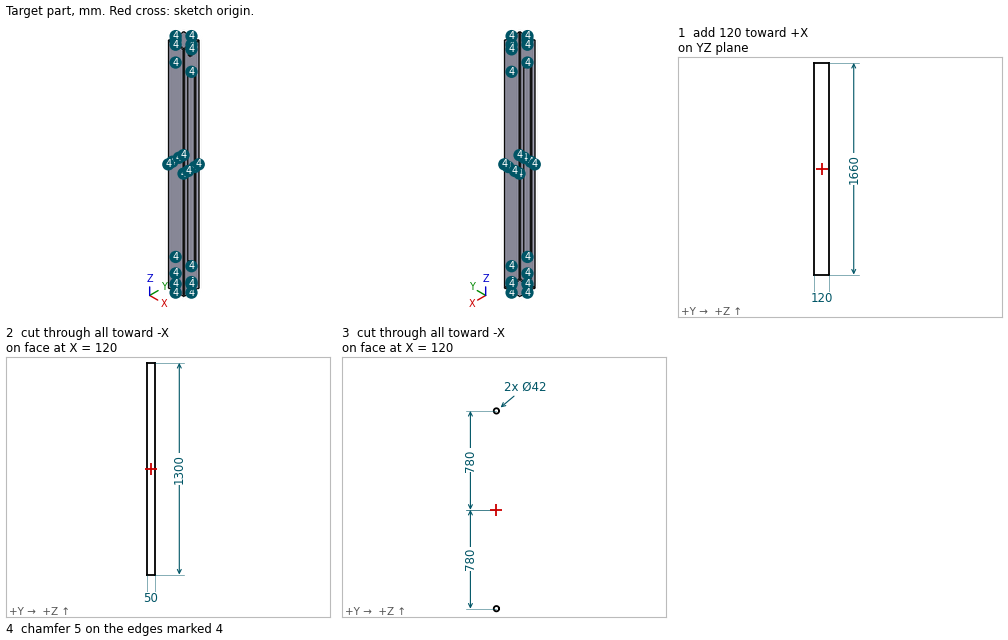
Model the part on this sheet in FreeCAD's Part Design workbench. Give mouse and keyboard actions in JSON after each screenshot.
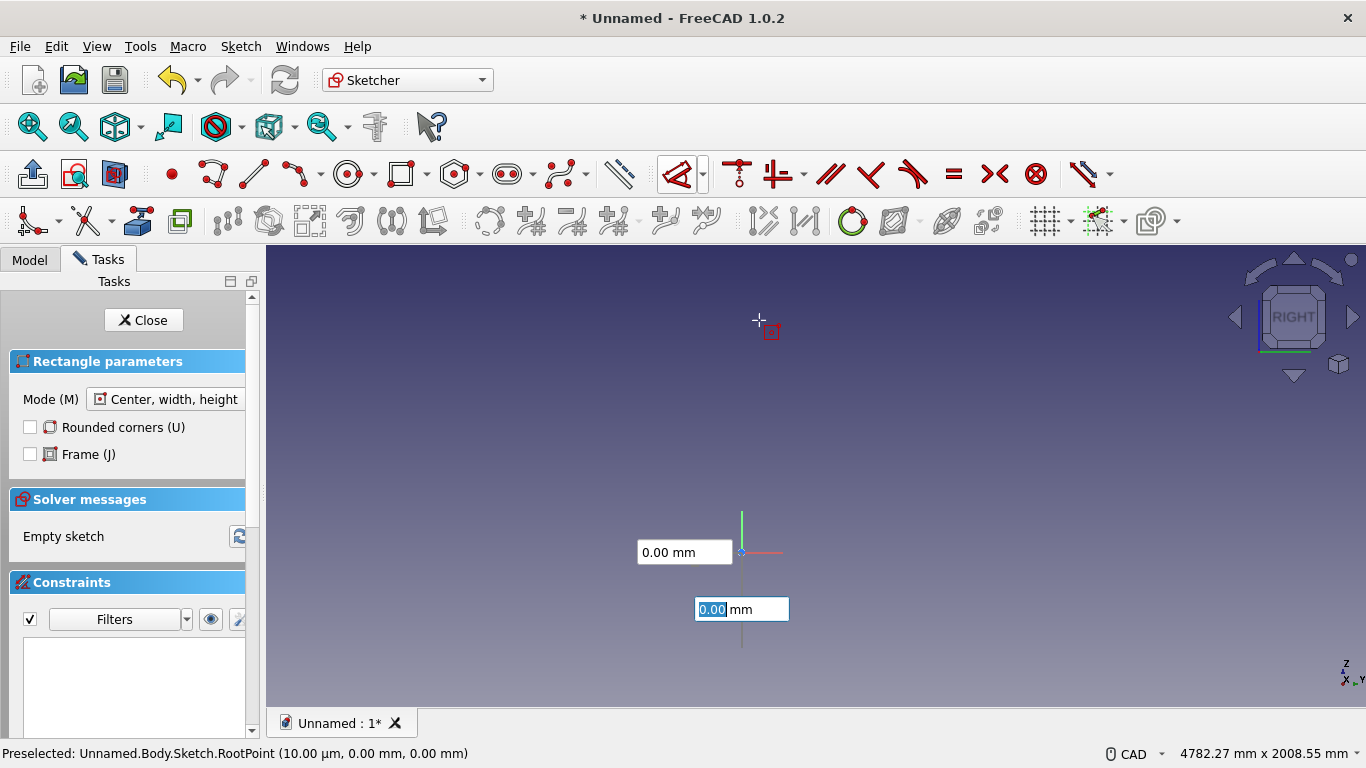
{"action": "left_click", "coordinate": [759, 320]}
{"action": "key", "text": "Escape"}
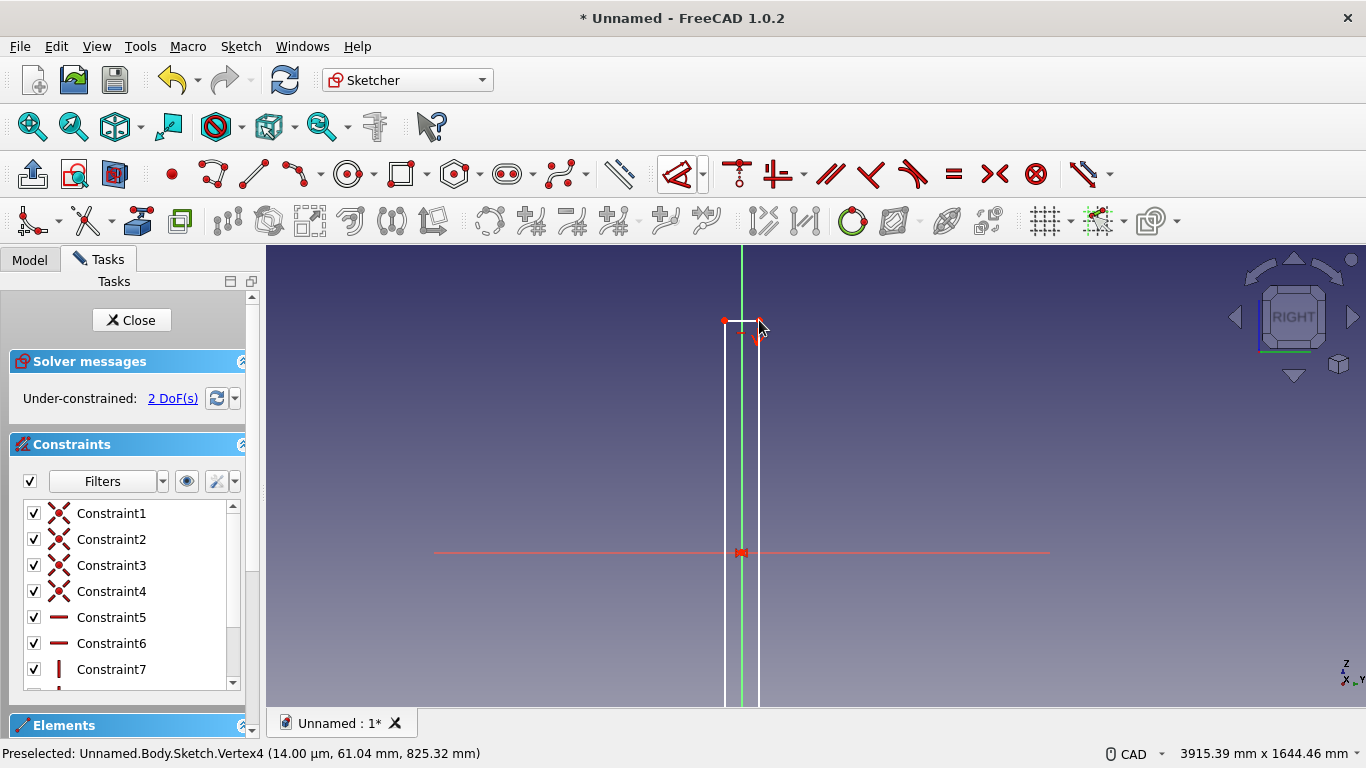
{"action": "key", "text": "d"}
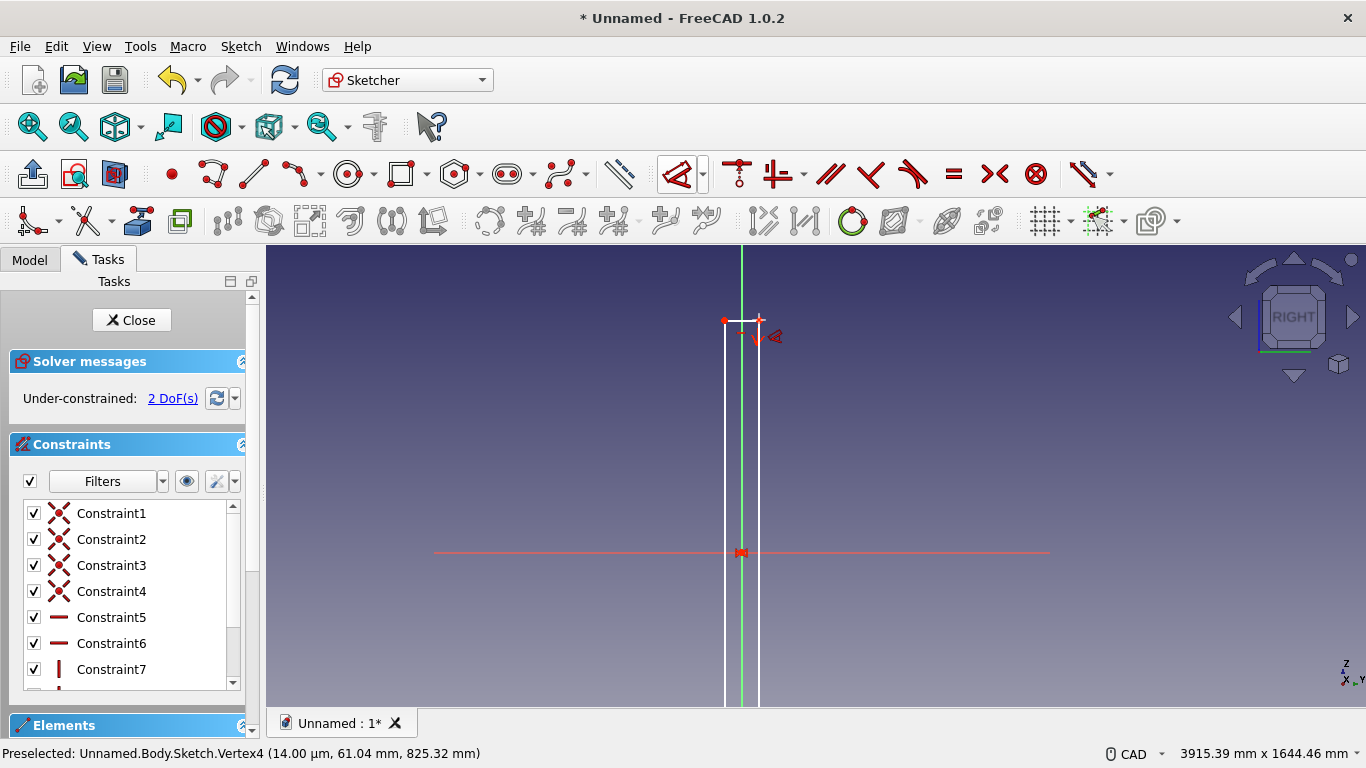
{"action": "scroll", "coordinate": [759, 320], "scroll_direction": "down", "scroll_amount": 2}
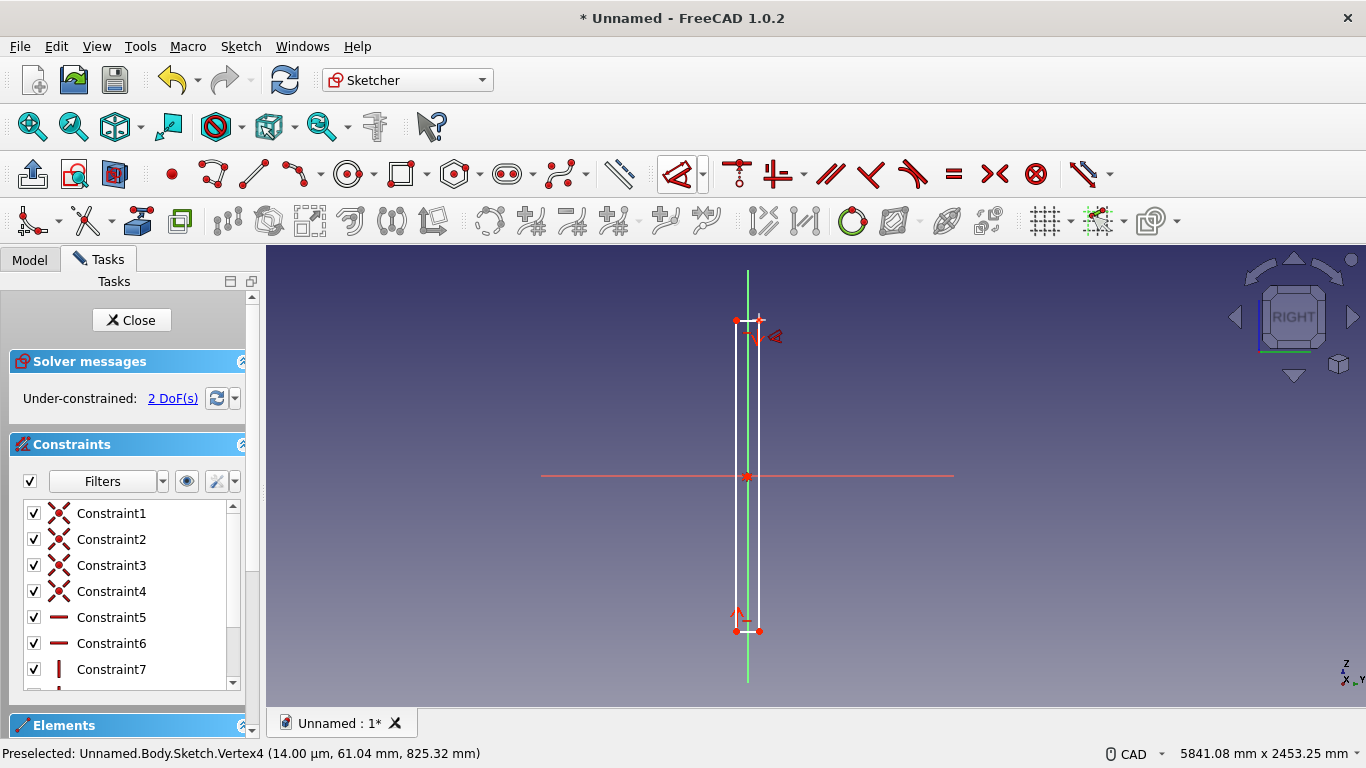
{"action": "scroll", "coordinate": [745, 632], "scroll_direction": "up", "scroll_amount": 3}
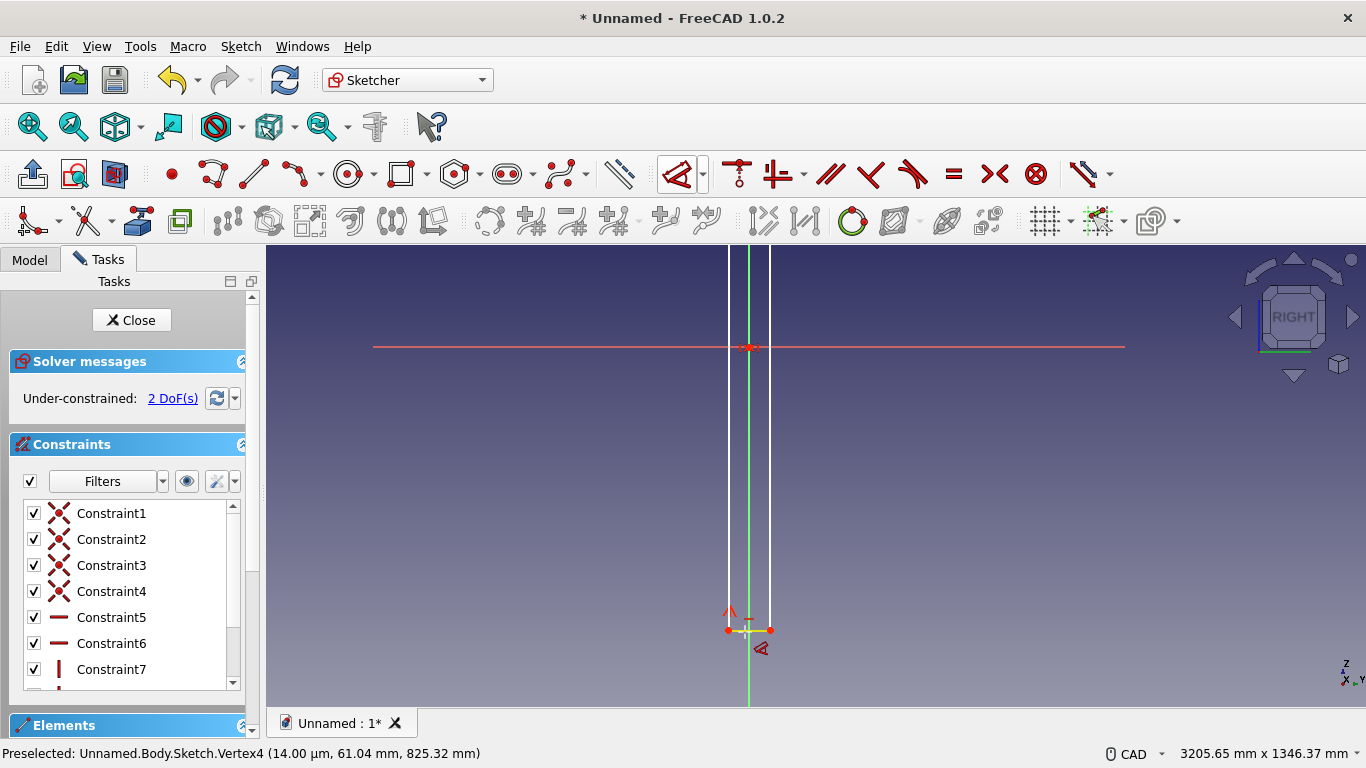
{"action": "left_click", "coordinate": [745, 631]}
{"action": "left_click", "coordinate": [735, 665]}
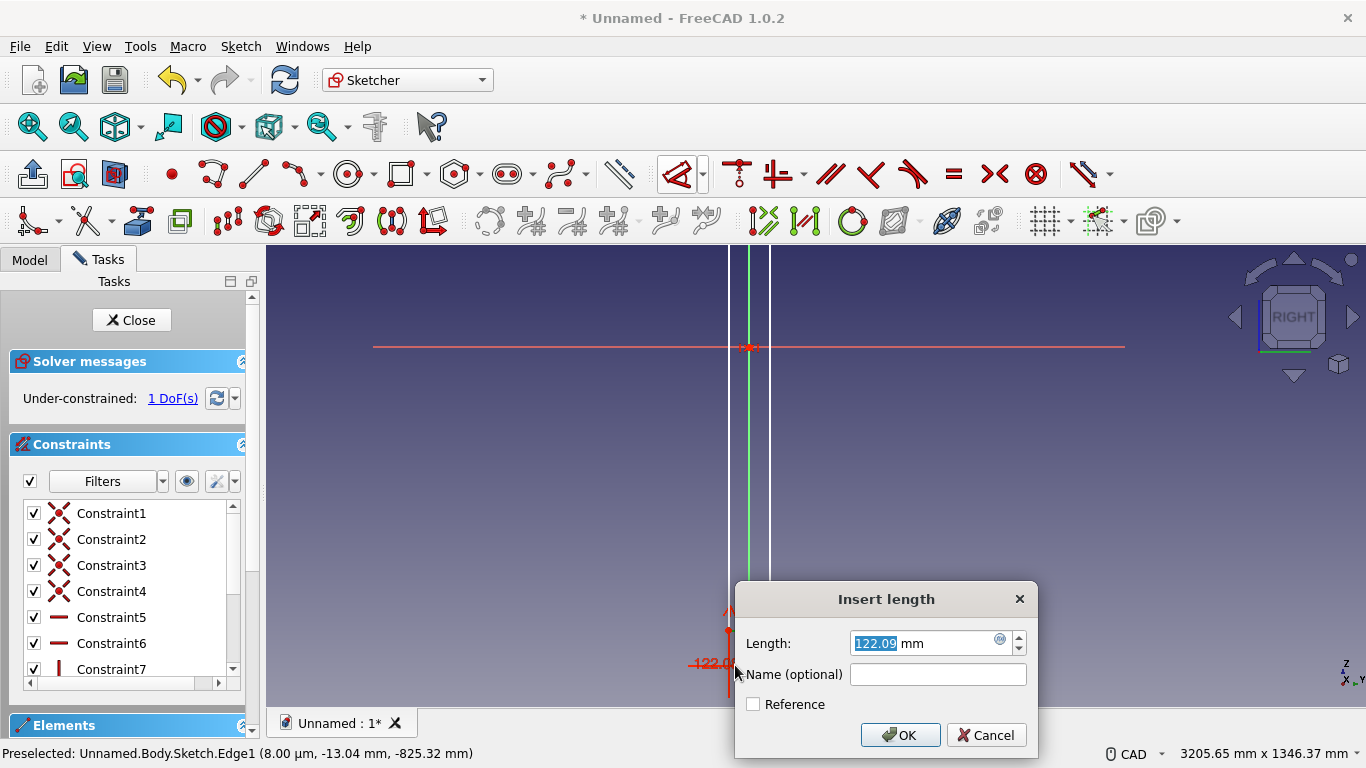
{"action": "type", "text": "120"}
{"action": "key", "text": "Return"}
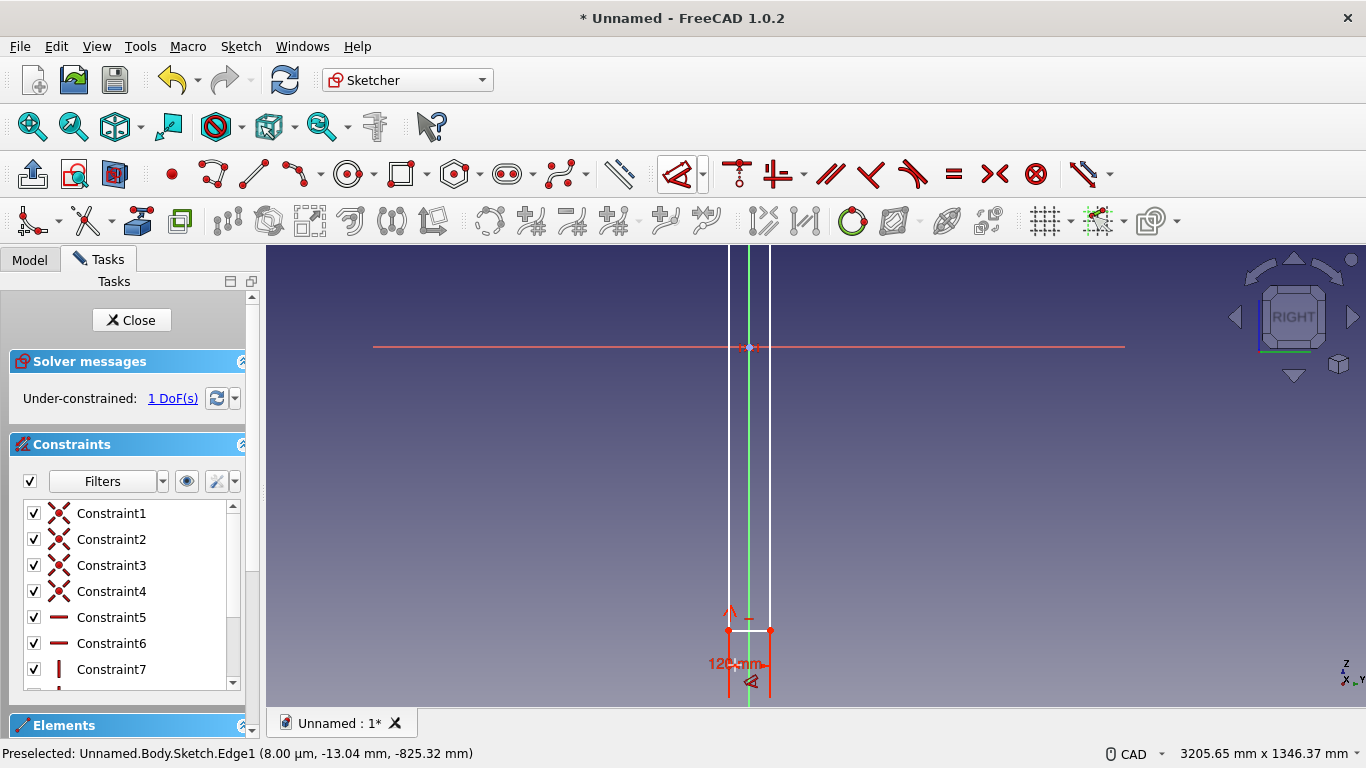
{"action": "left_click", "coordinate": [770, 461]}
{"action": "left_click", "coordinate": [804, 452]}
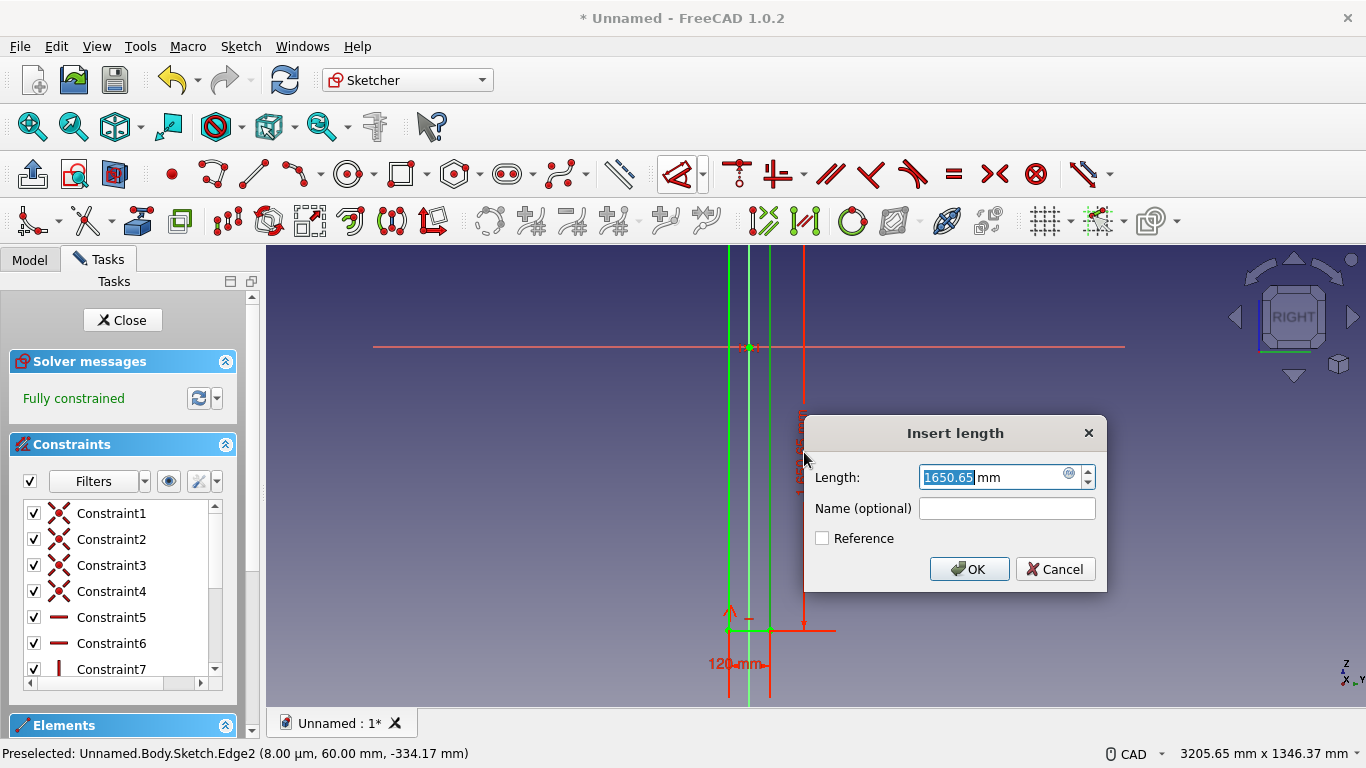
{"action": "type", "text": "1660"}
{"action": "key", "text": "Return"}
{"action": "key", "text": "Escape"}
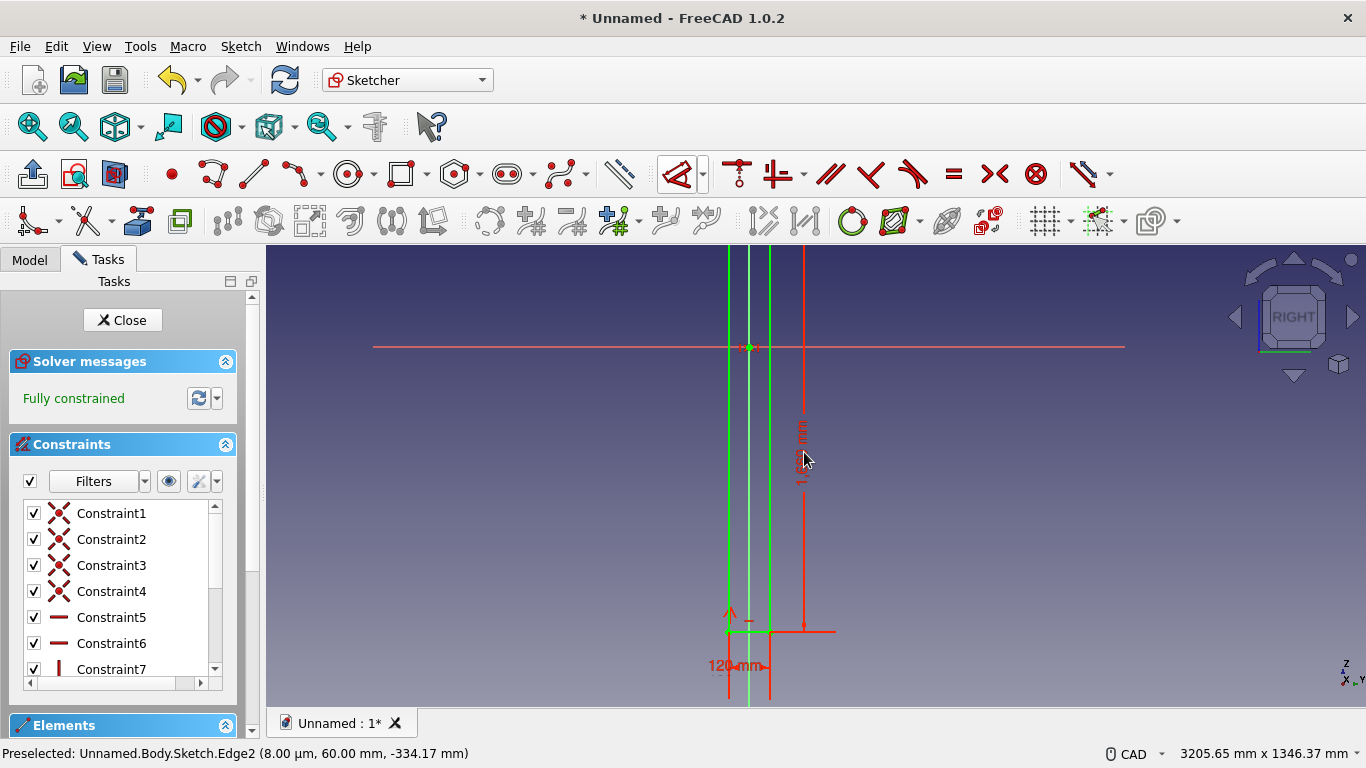
{"action": "left_click", "coordinate": [123, 320]}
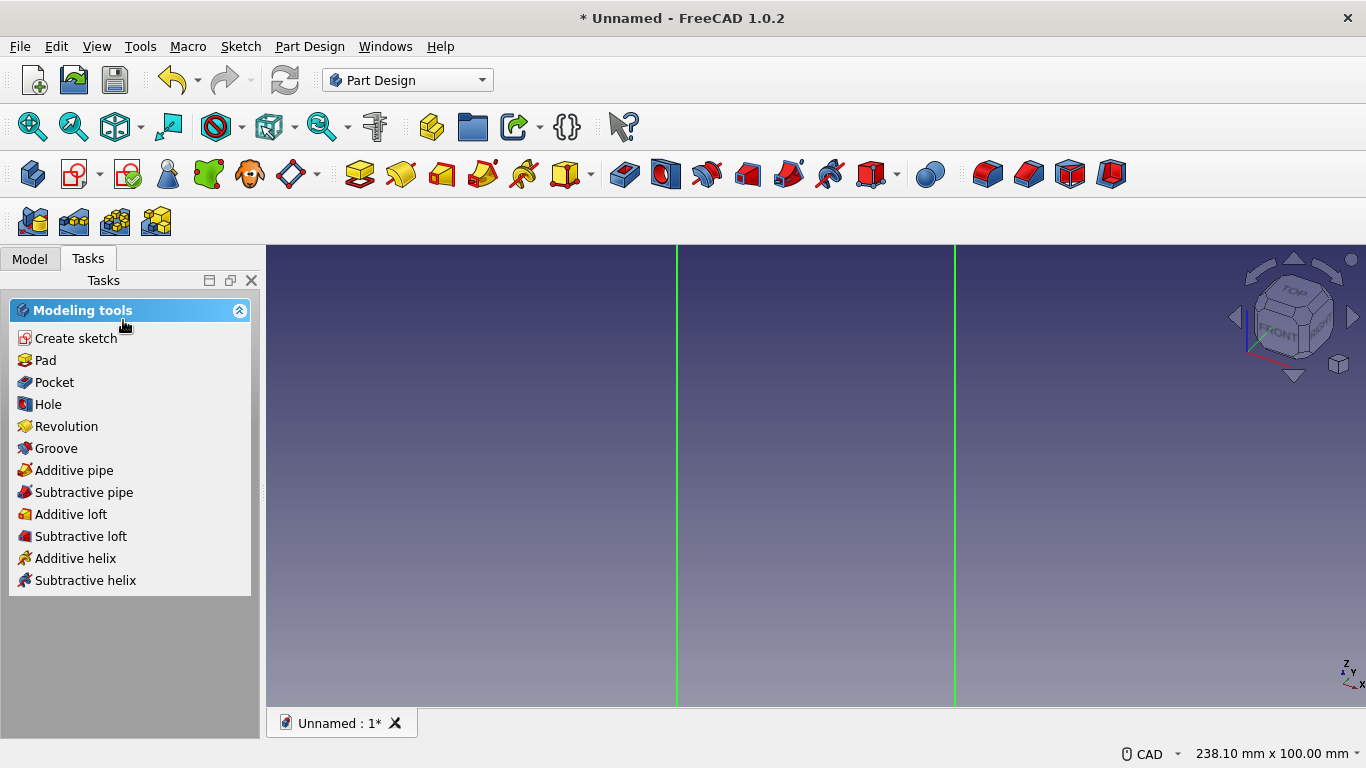
{"action": "left_click", "coordinate": [360, 174]}